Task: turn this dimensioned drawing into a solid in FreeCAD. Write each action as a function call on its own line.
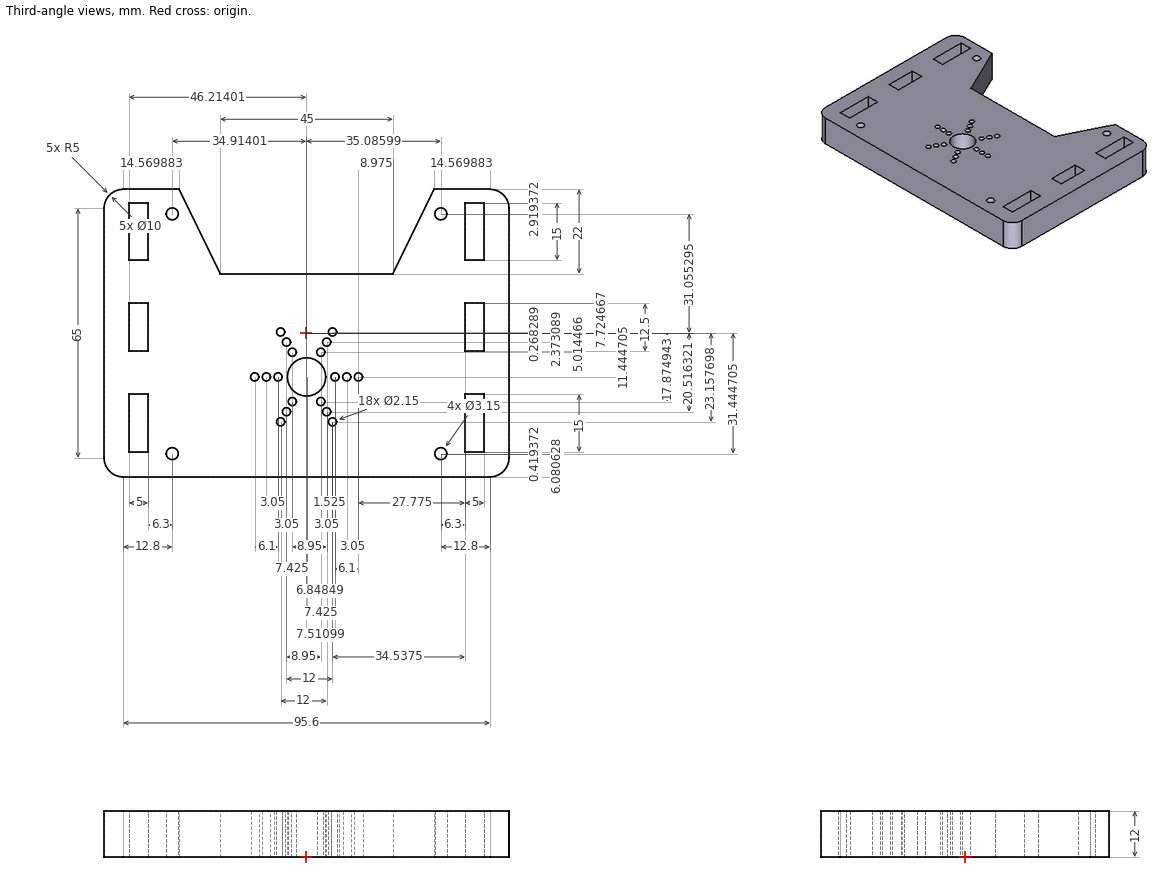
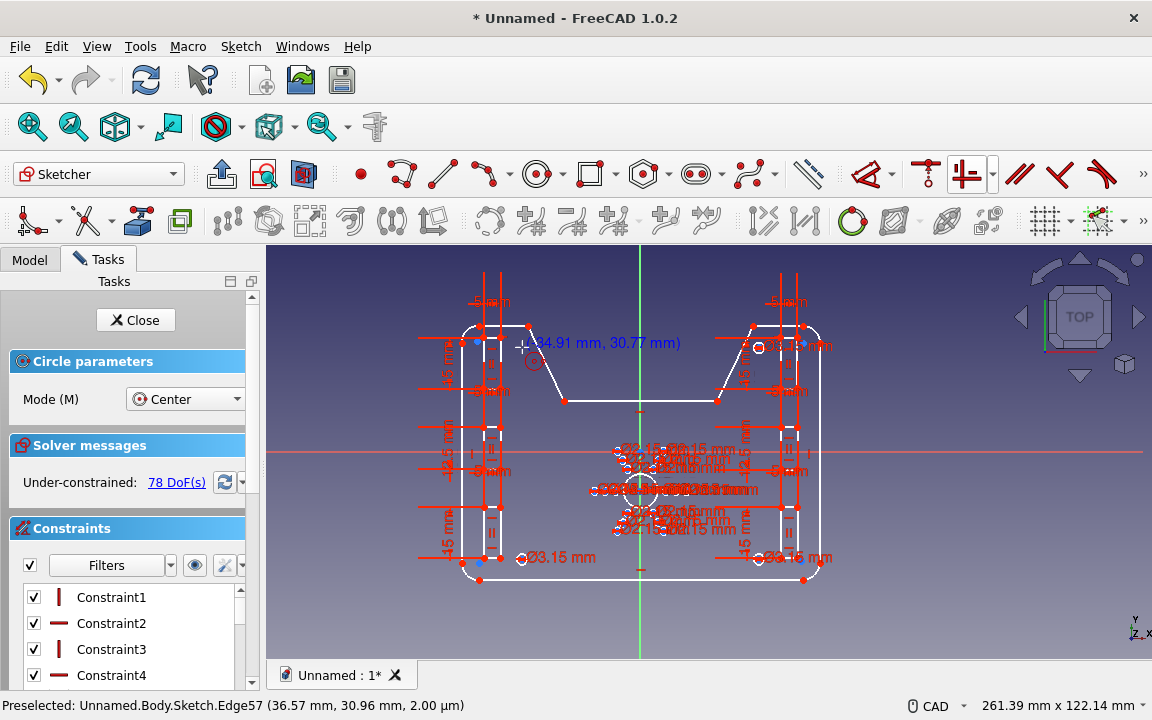
click(522, 347)
move(518, 343)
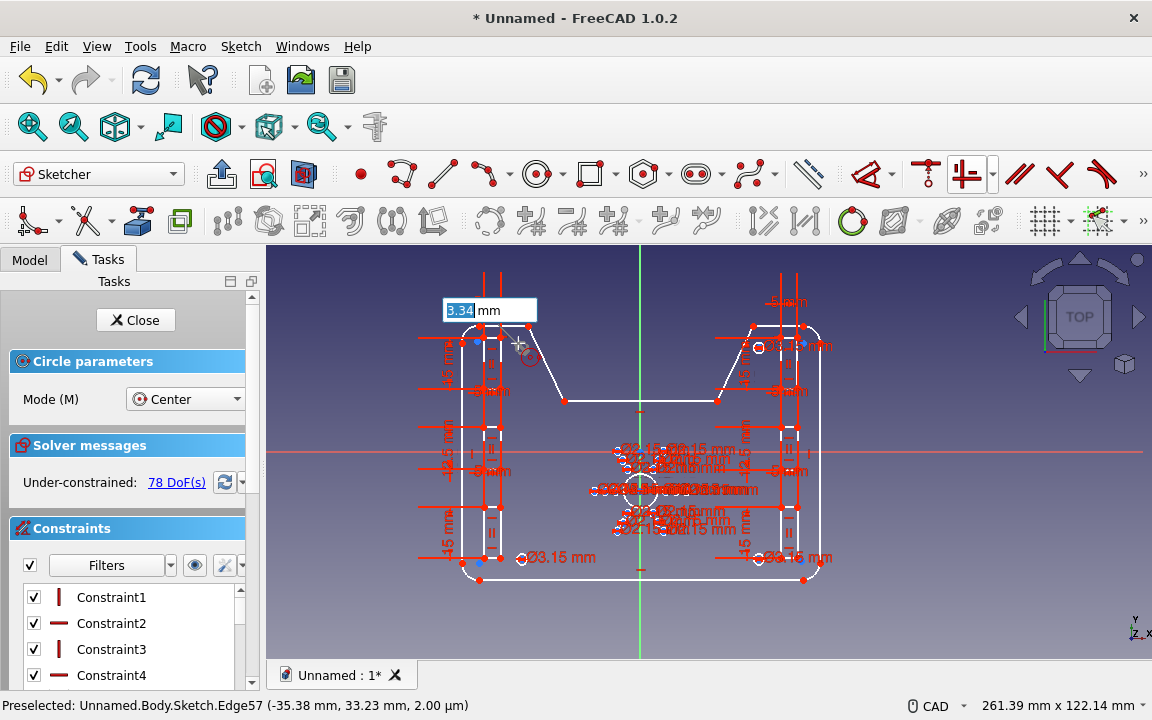
text(3.15)
key(Return)
key(Escape)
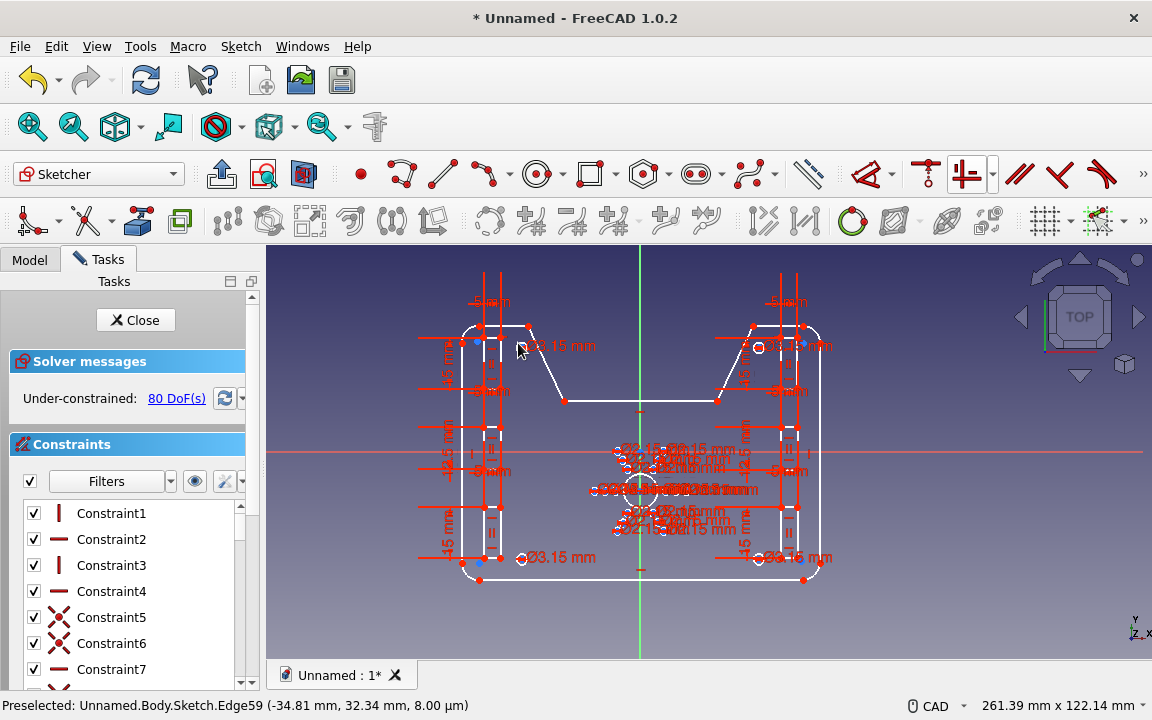
click(462, 409)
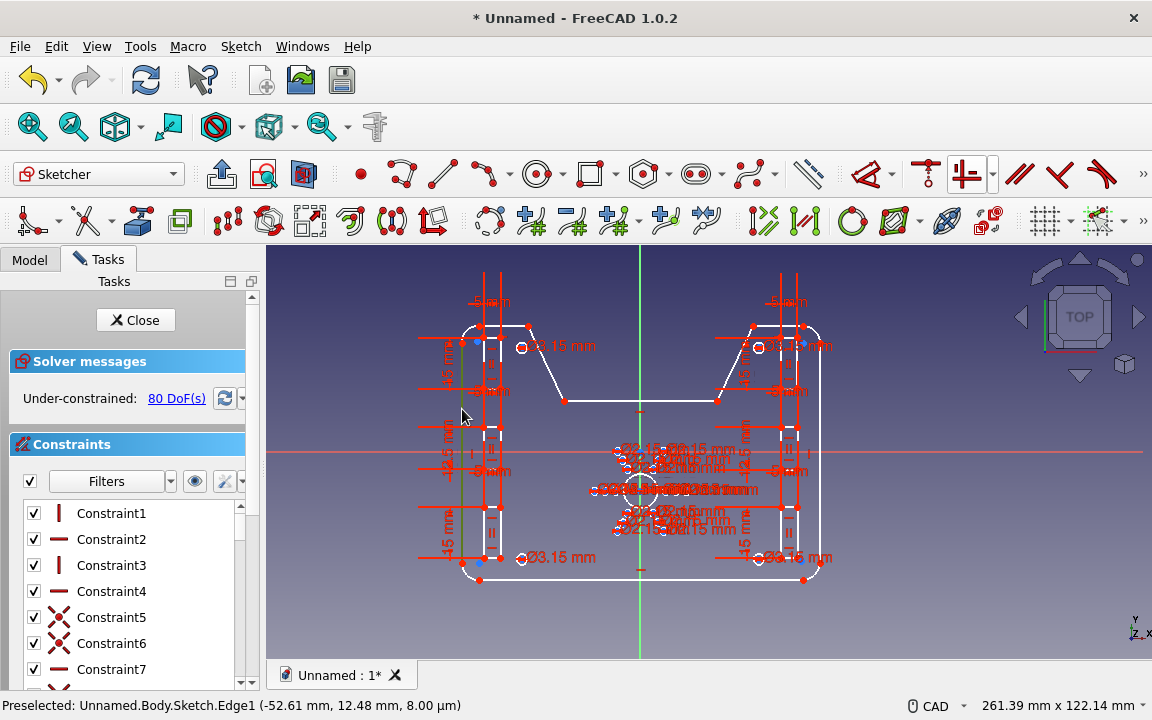
click(467, 575)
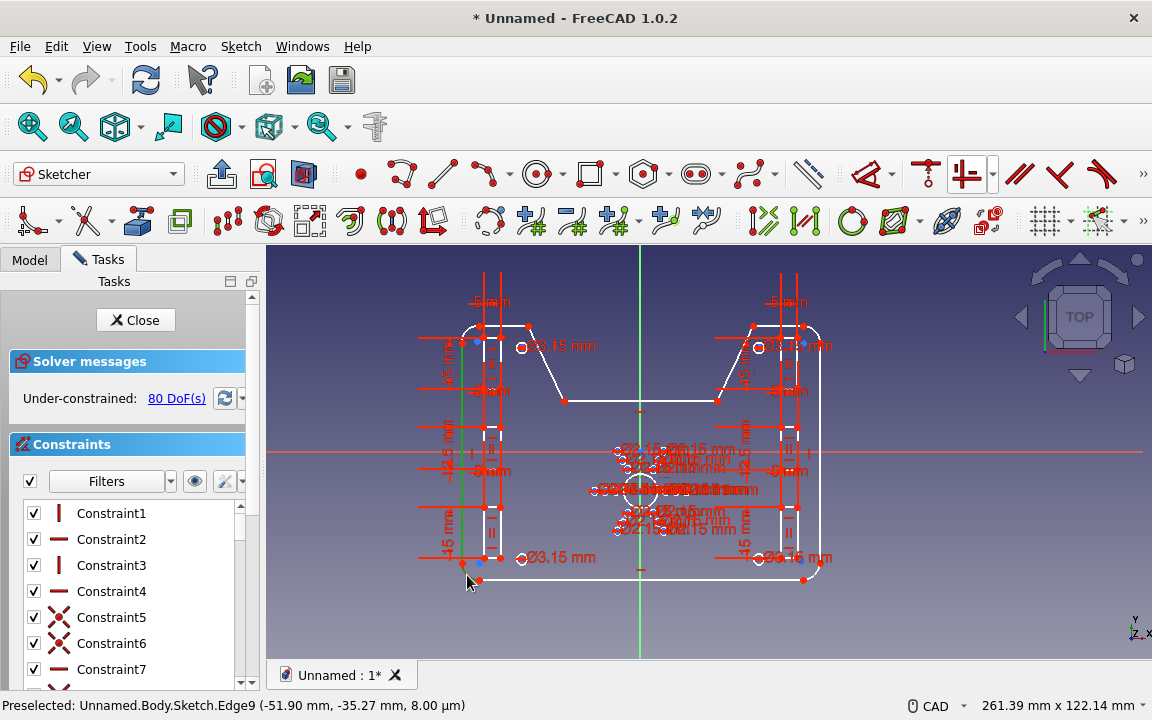
key(t)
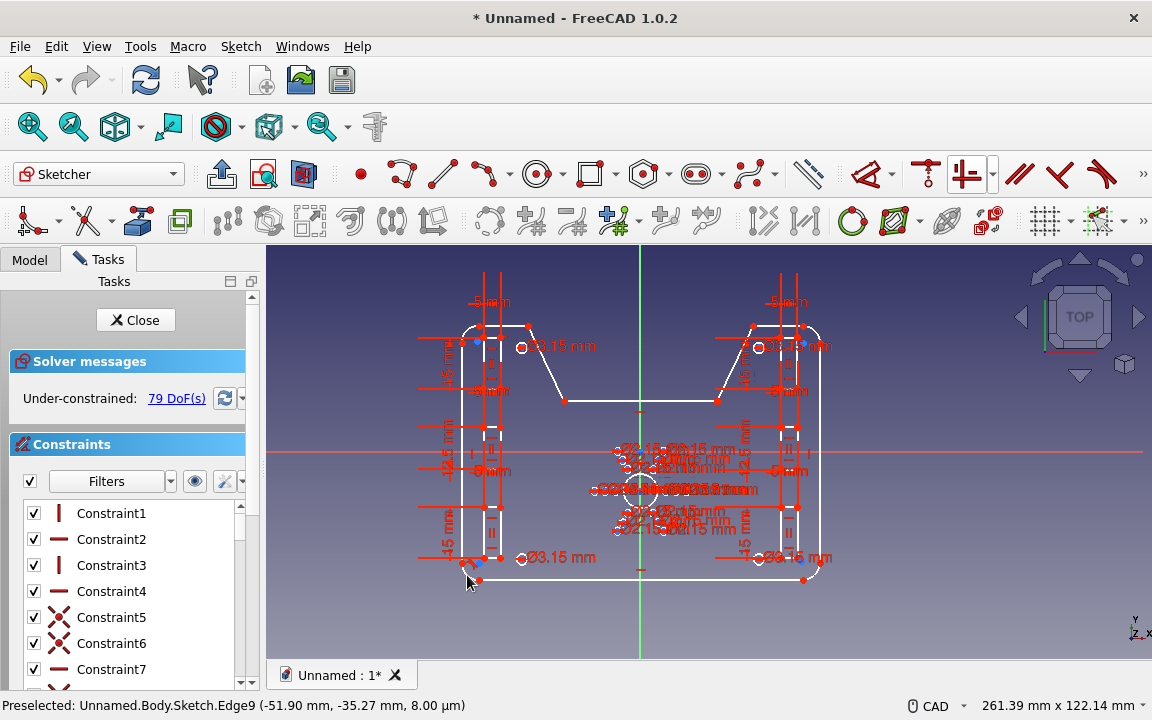
click(462, 409)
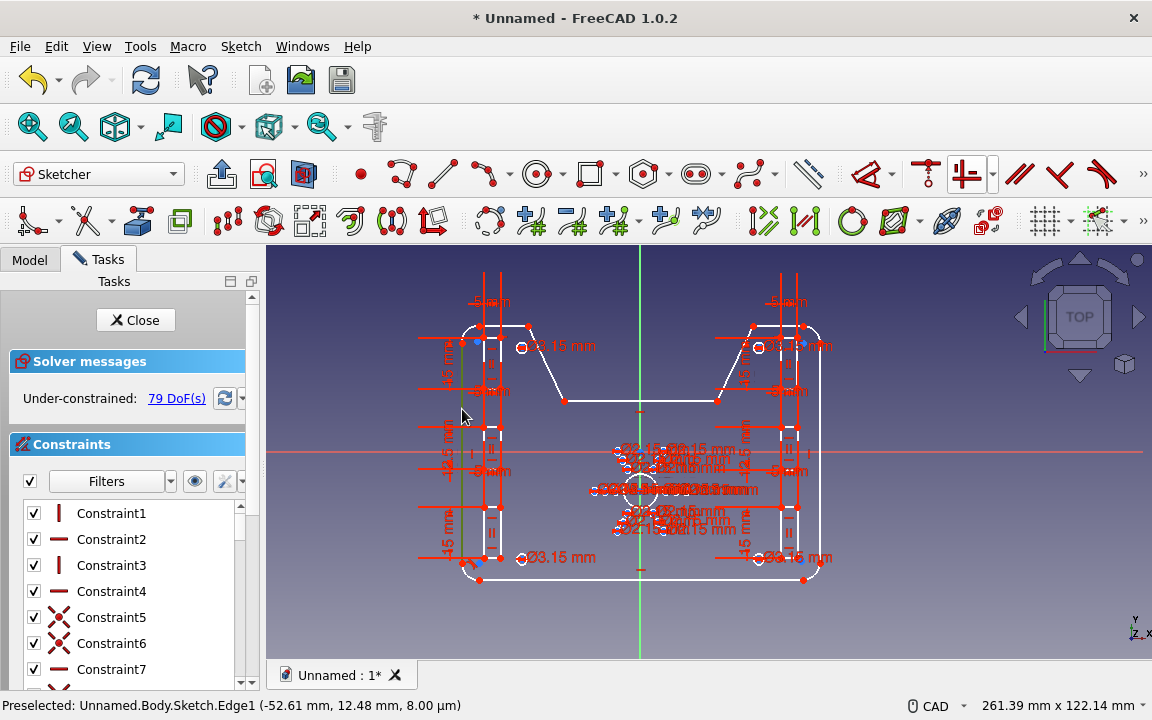
click(467, 331)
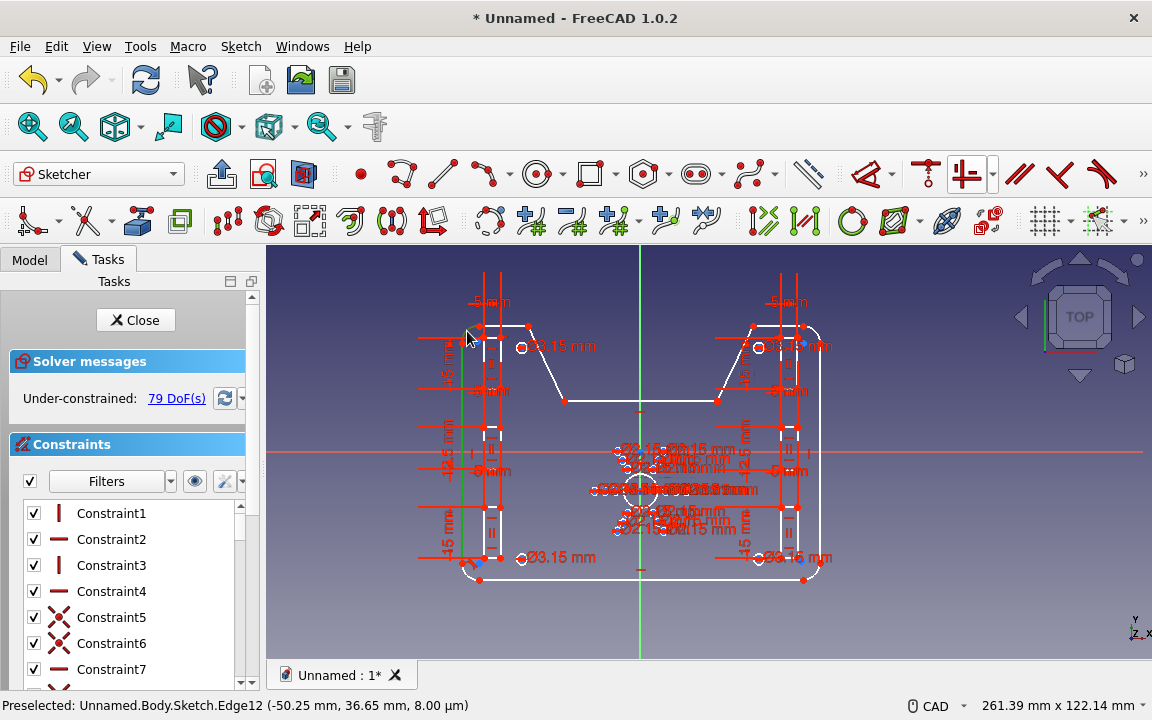
key(t)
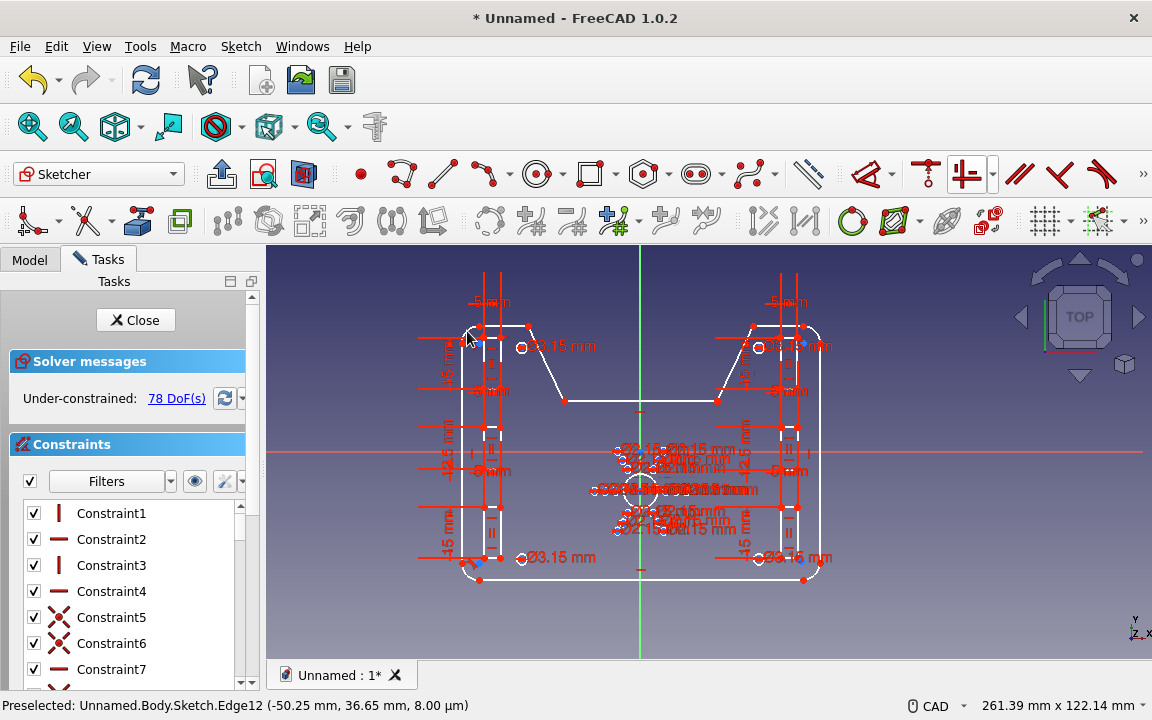
click(576, 580)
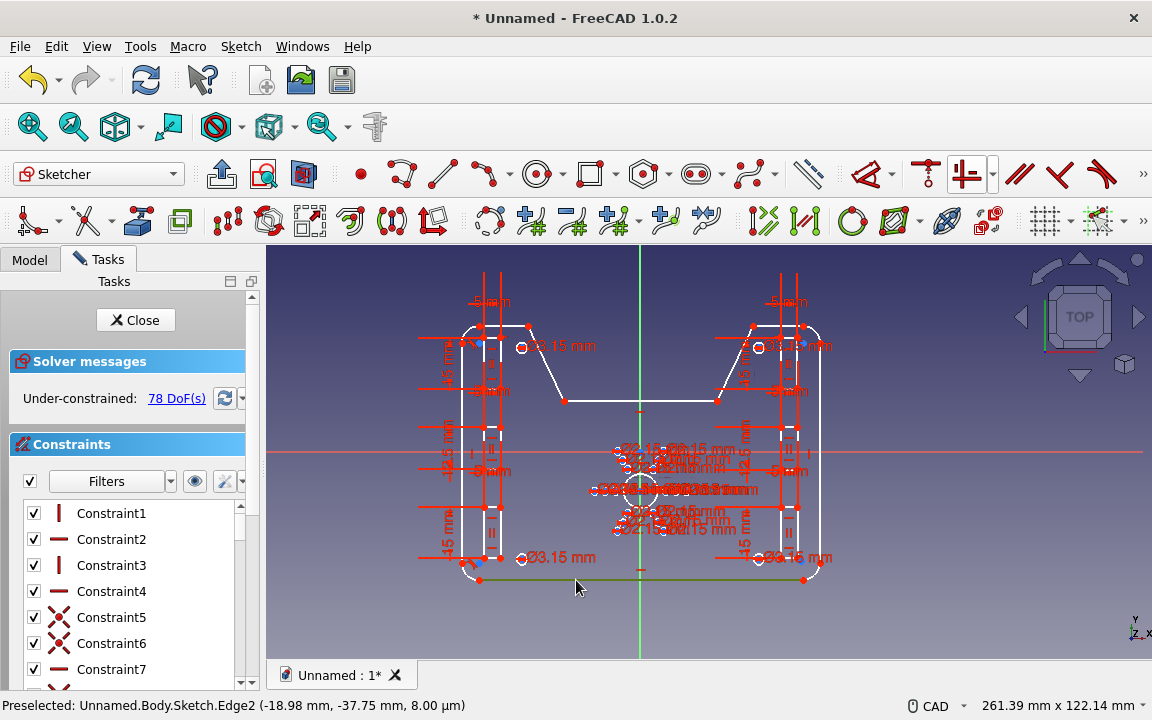
click(467, 575)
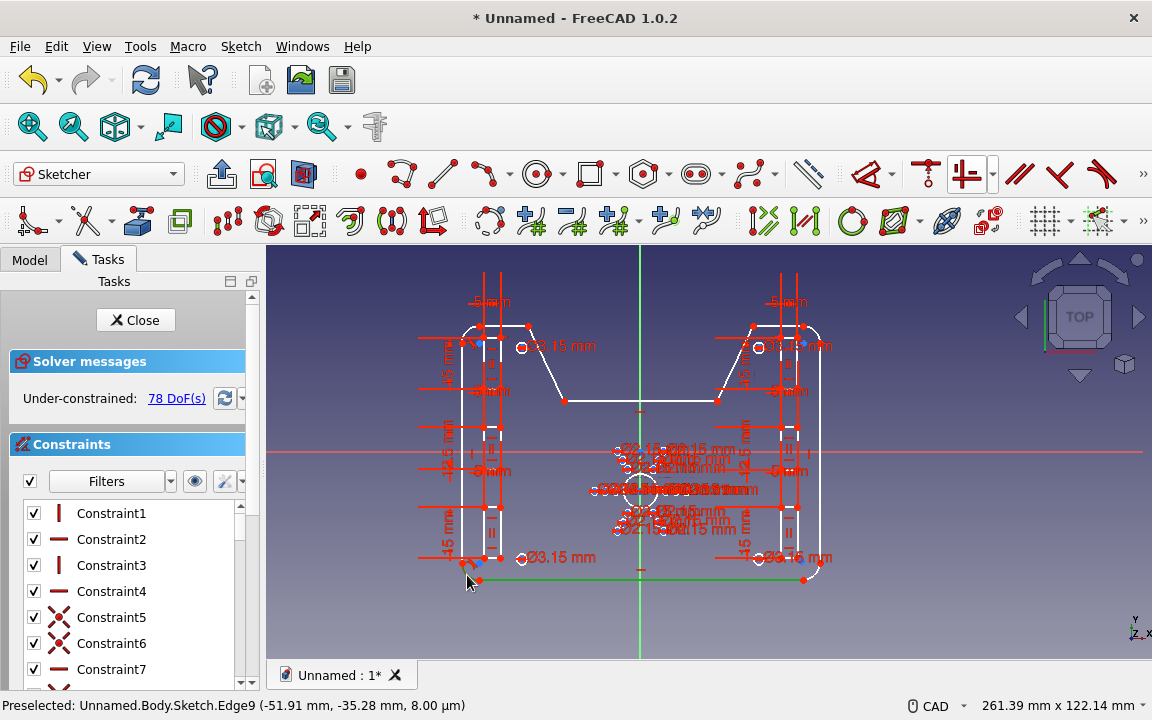
key(t)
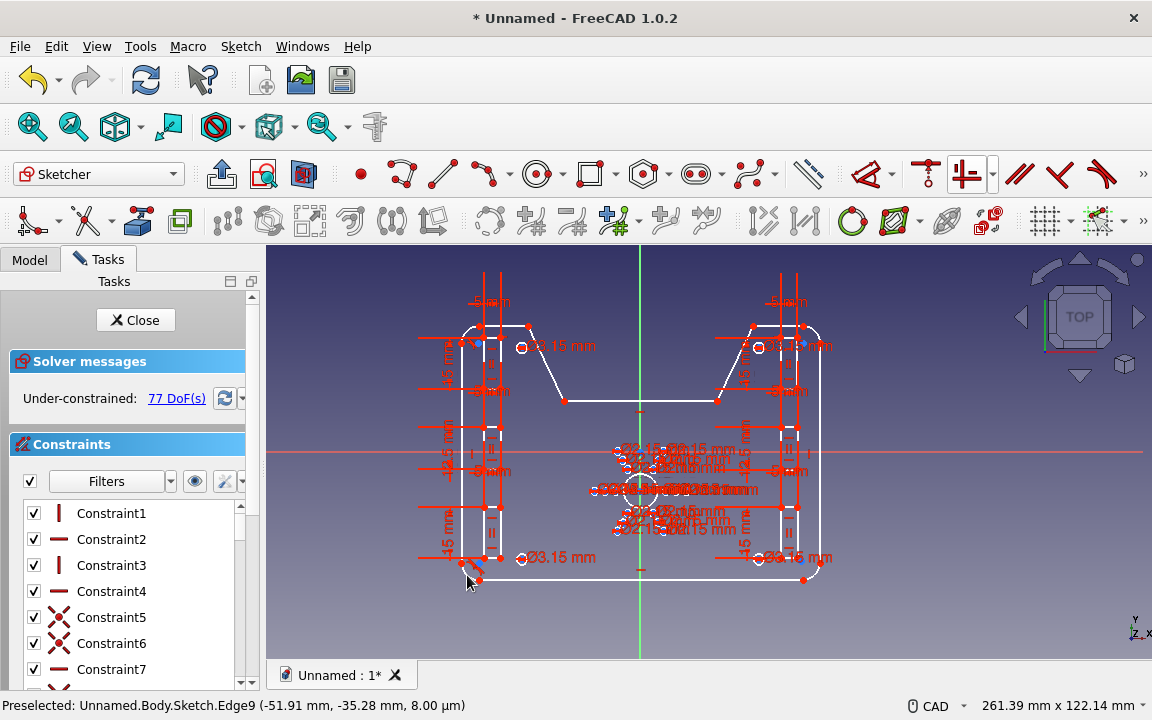
click(576, 580)